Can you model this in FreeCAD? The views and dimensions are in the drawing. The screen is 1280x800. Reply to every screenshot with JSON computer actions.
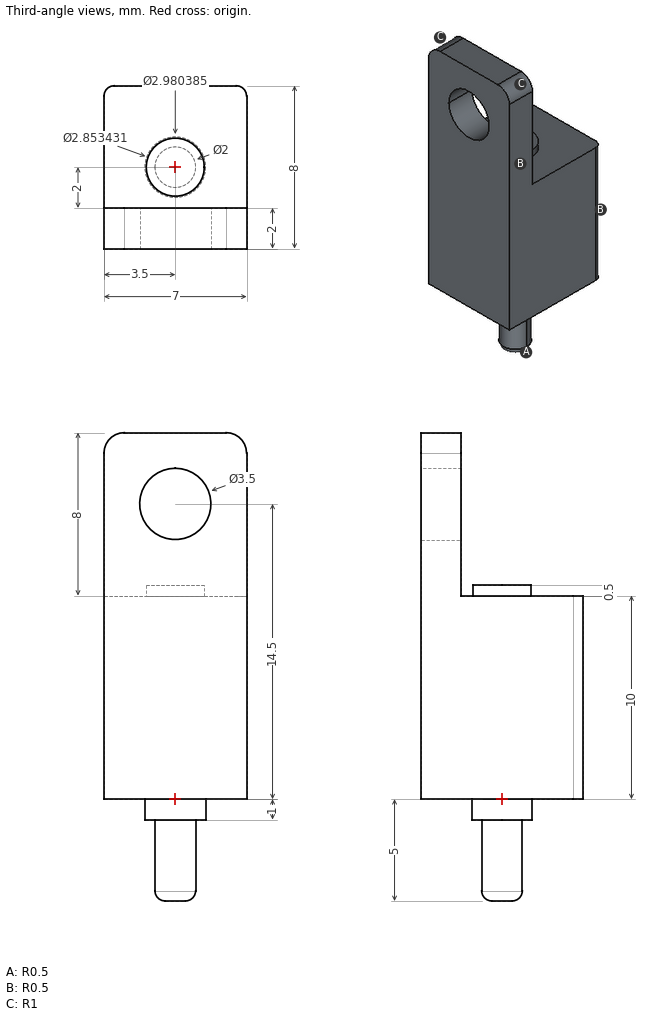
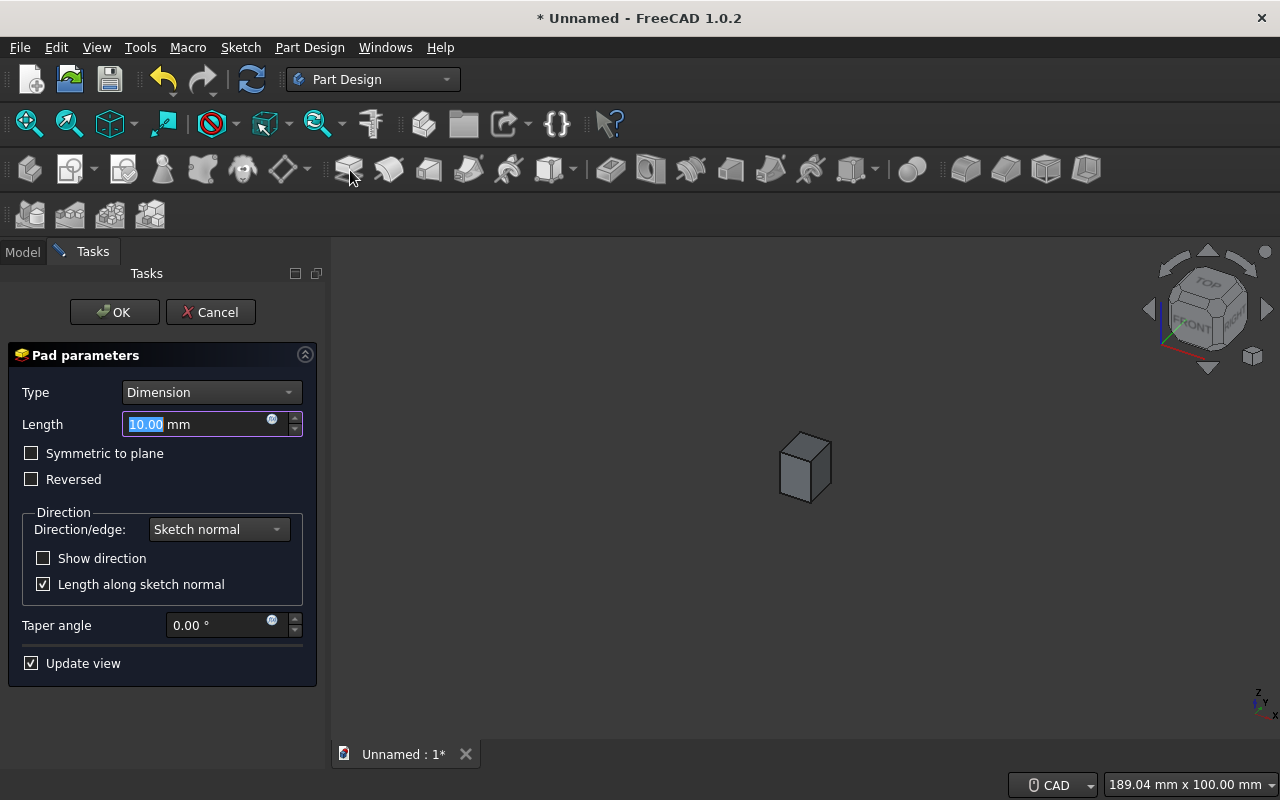
{"action": "type", "text": "10"}
{"action": "key", "text": "Tab"}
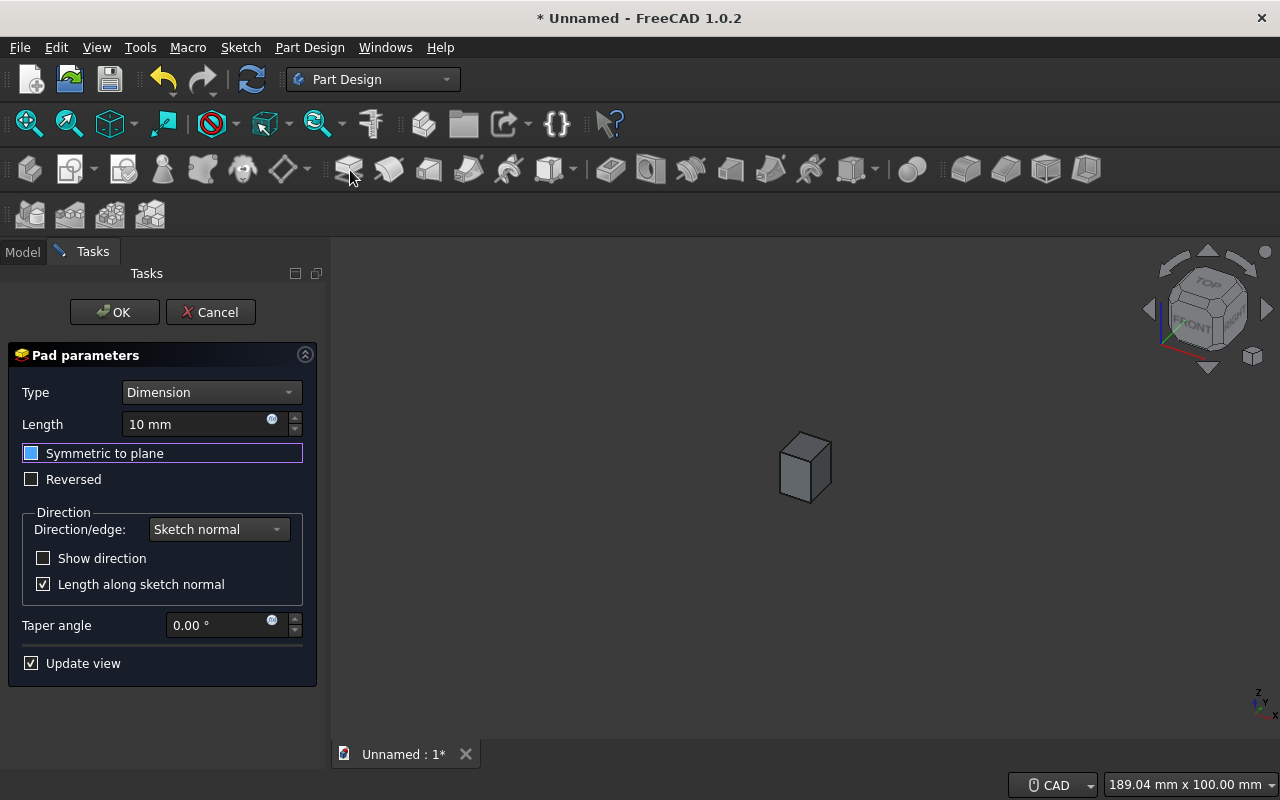
{"action": "left_click", "coordinate": [115, 312]}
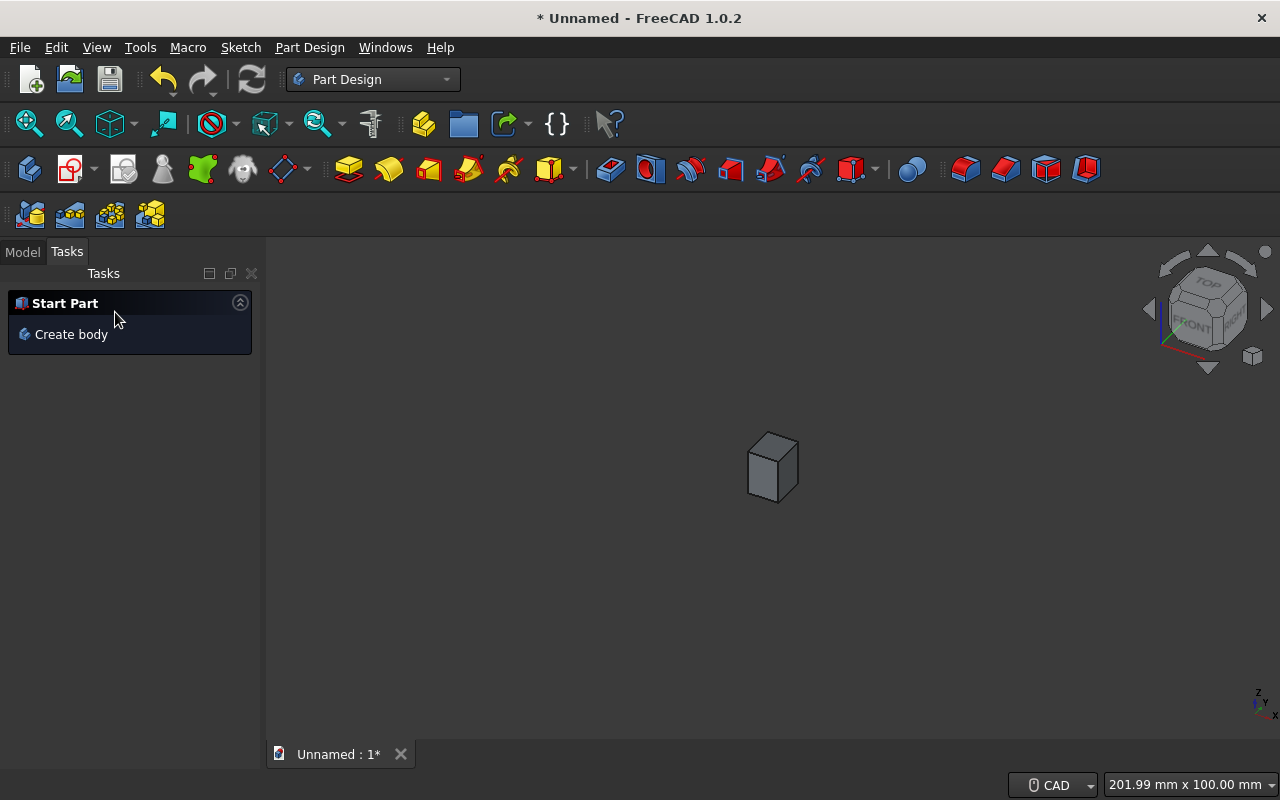
{"action": "key", "text": "v f"}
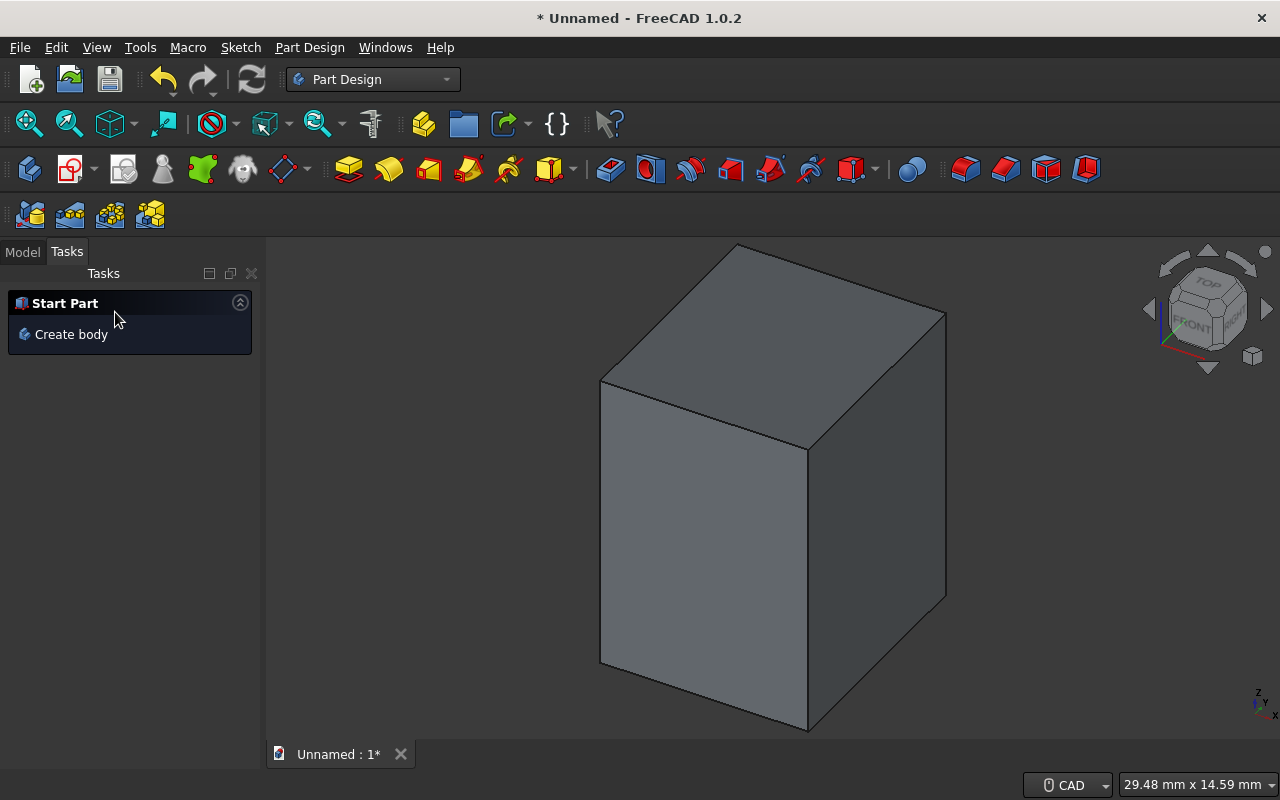
{"action": "left_click", "coordinate": [773, 346]}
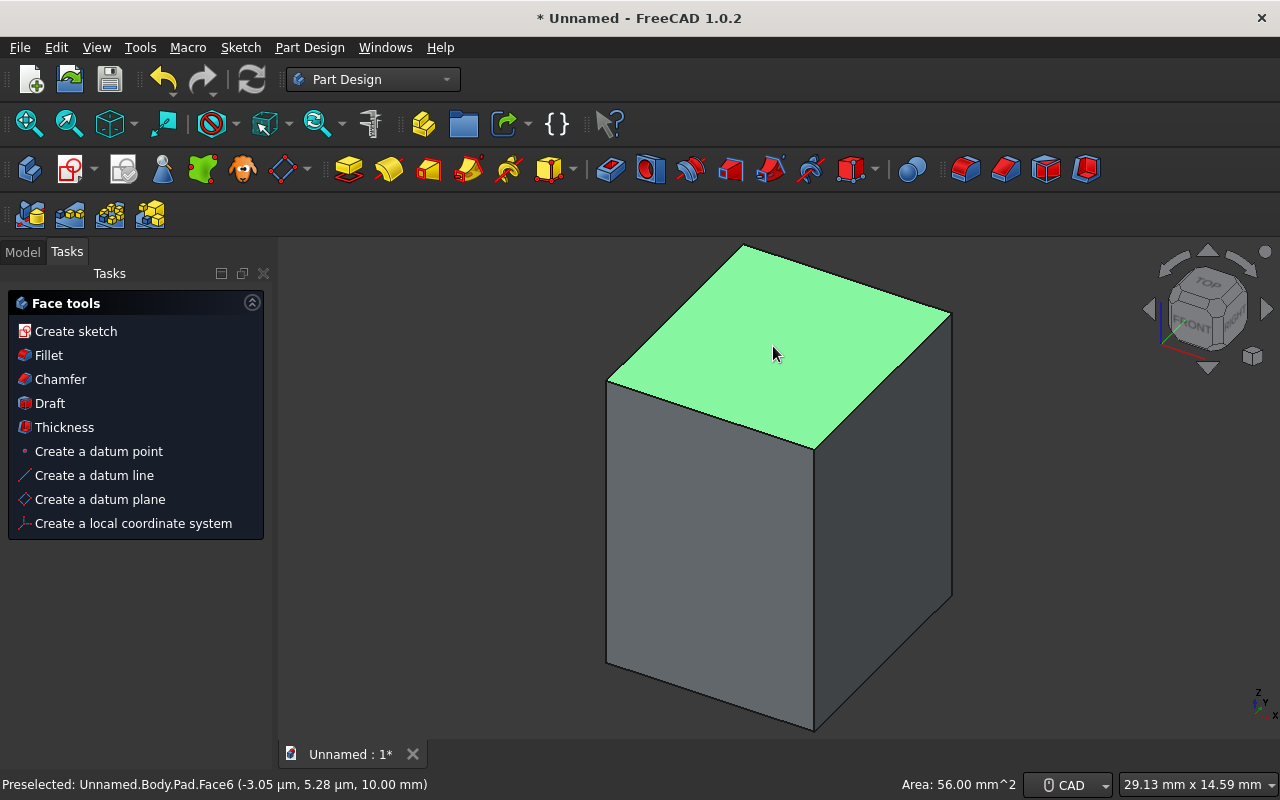
{"action": "left_click", "coordinate": [70, 170]}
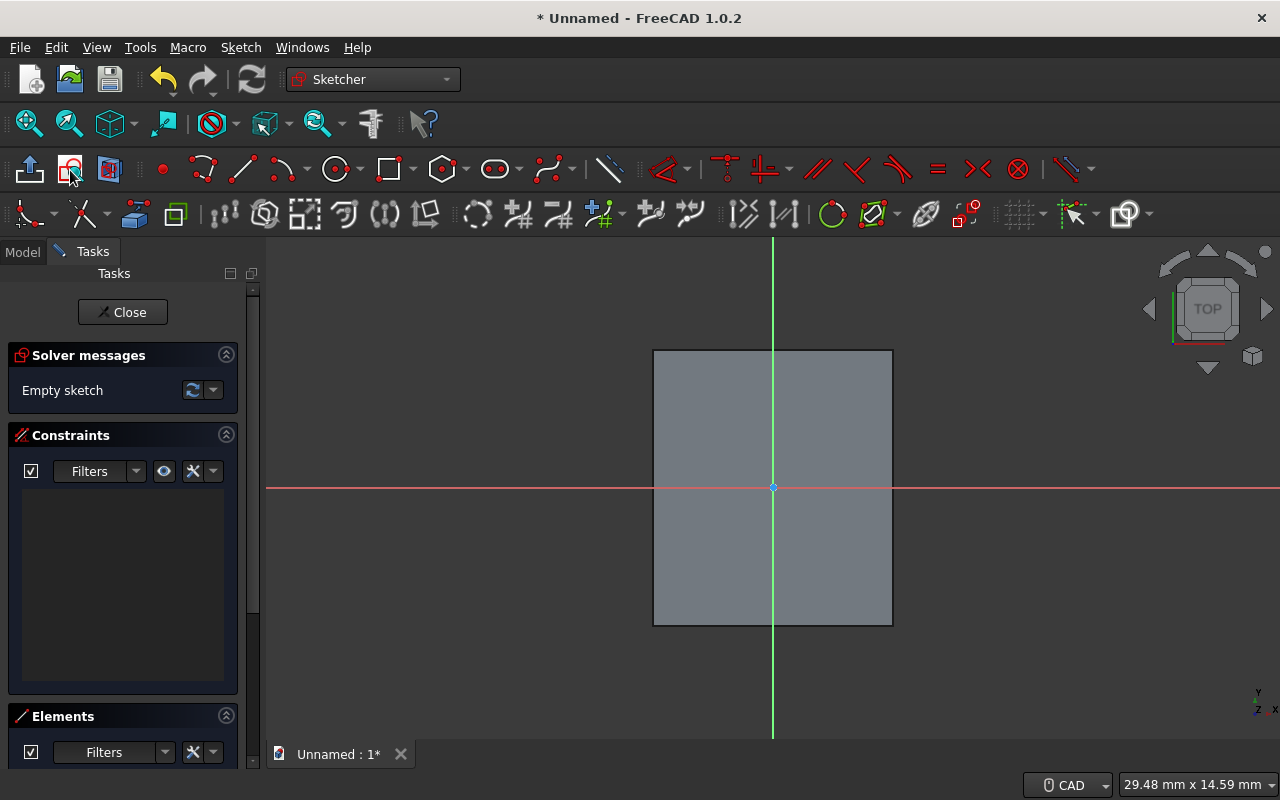
{"action": "scroll", "coordinate": [829, 613], "scroll_direction": "up", "scroll_amount": 4}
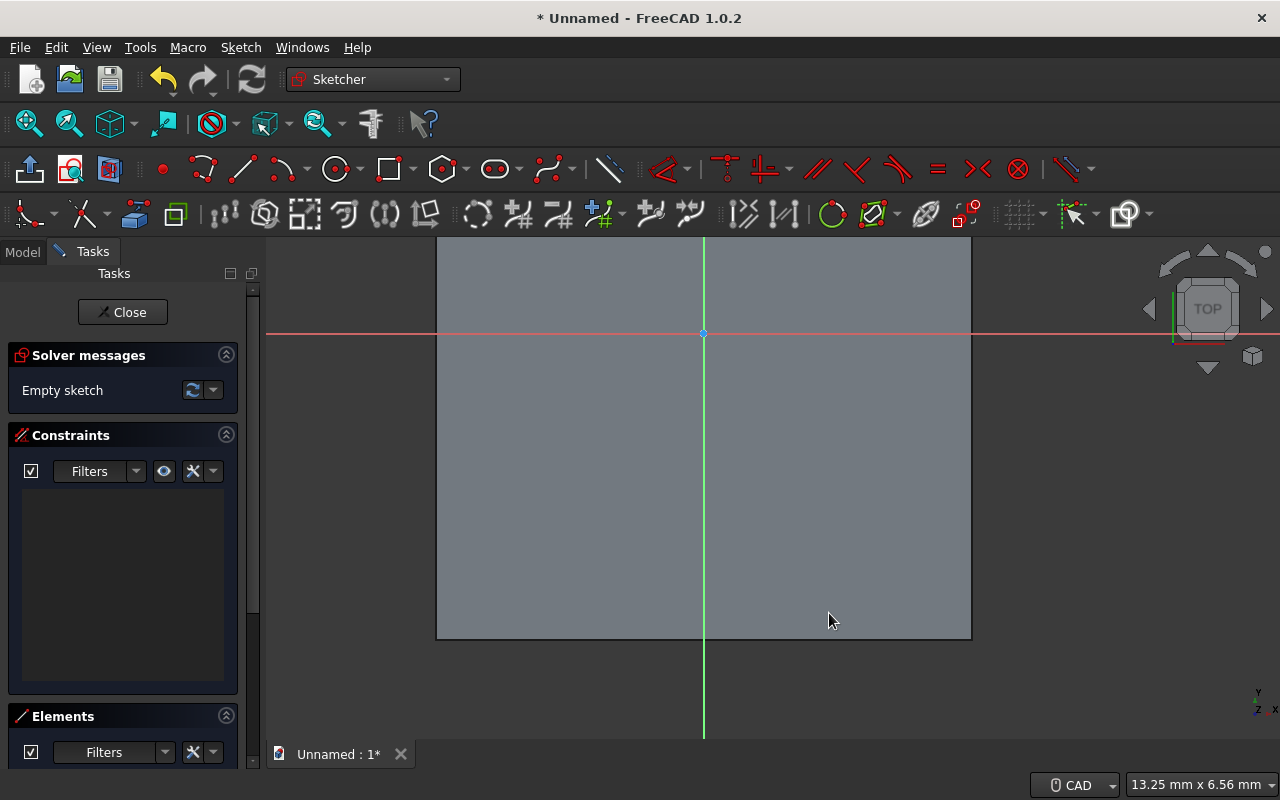
{"action": "key", "text": "g r"}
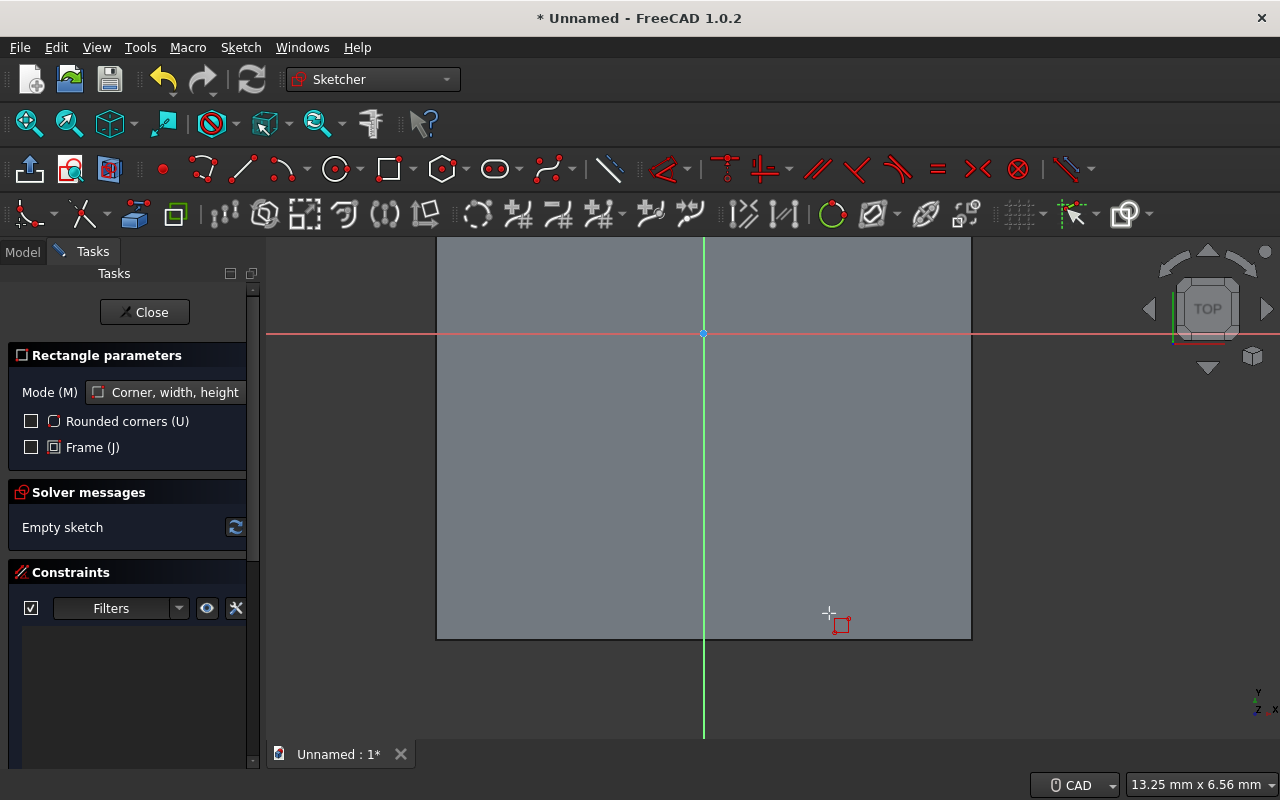
{"action": "left_click", "coordinate": [436, 487]}
{"action": "mouse_move", "coordinate": [972, 640]}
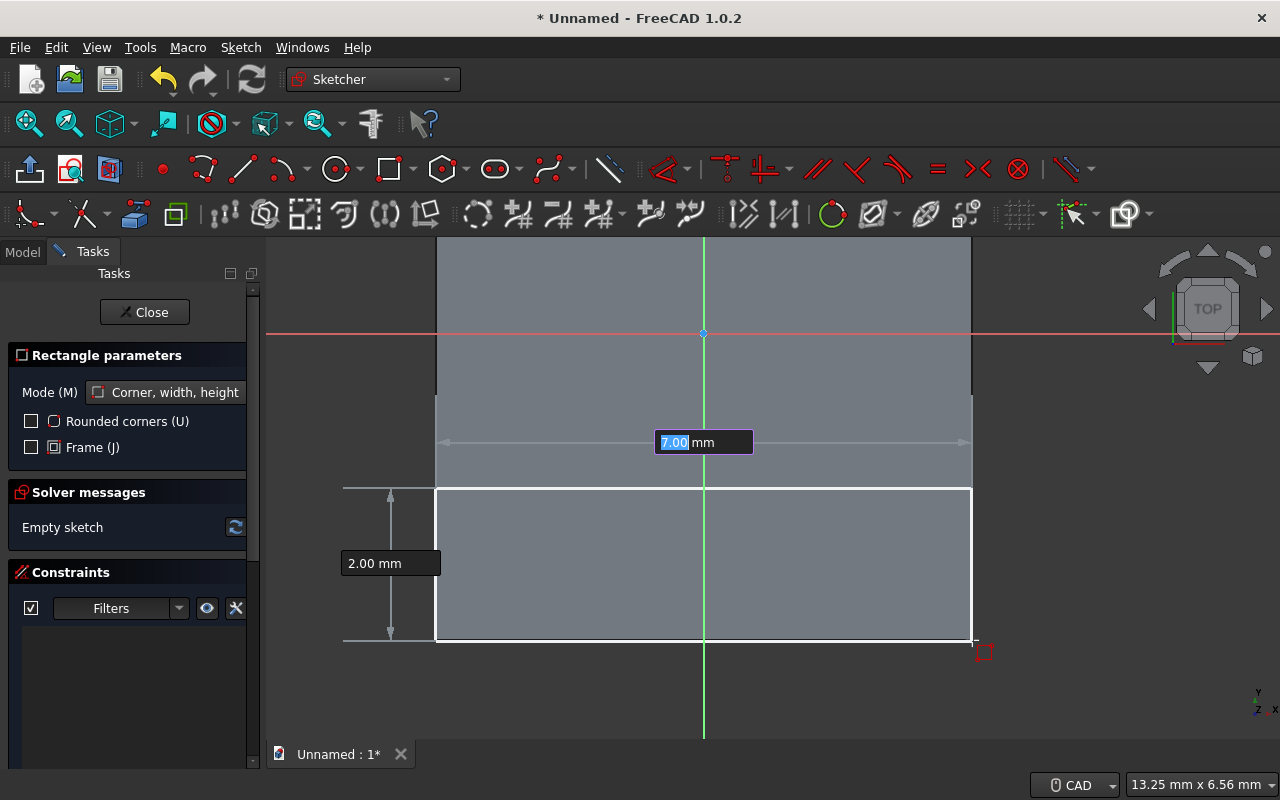
{"action": "type", "text": "7"}
{"action": "key", "text": "Tab"}
{"action": "type", "text": "2"}
{"action": "key", "text": "Return"}
{"action": "key", "text": "Escape"}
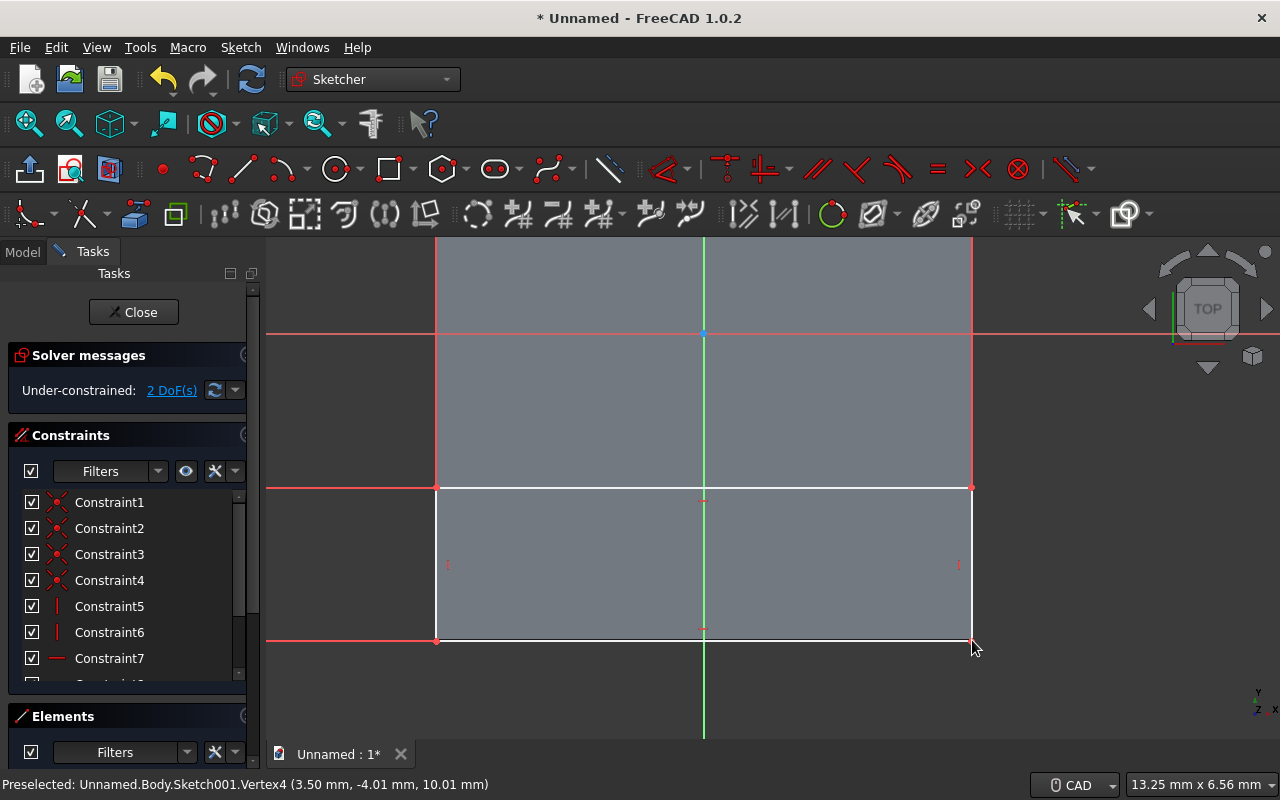
{"action": "key", "text": "d"}